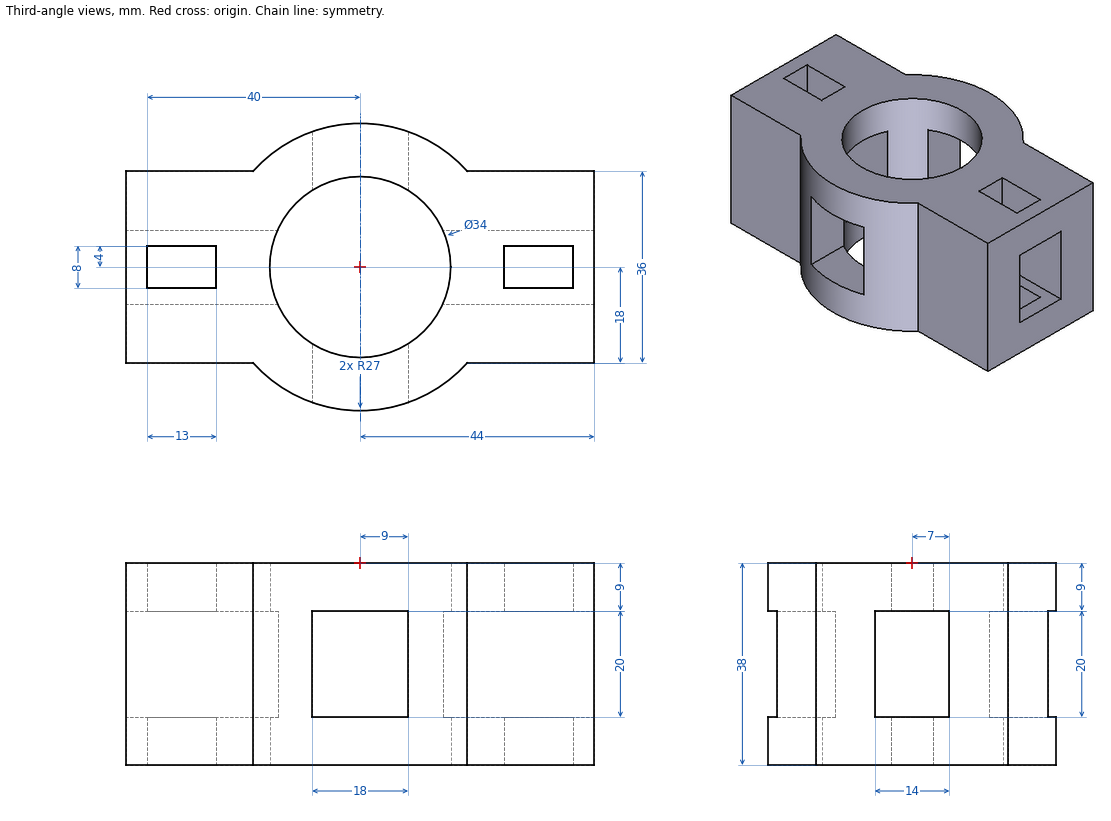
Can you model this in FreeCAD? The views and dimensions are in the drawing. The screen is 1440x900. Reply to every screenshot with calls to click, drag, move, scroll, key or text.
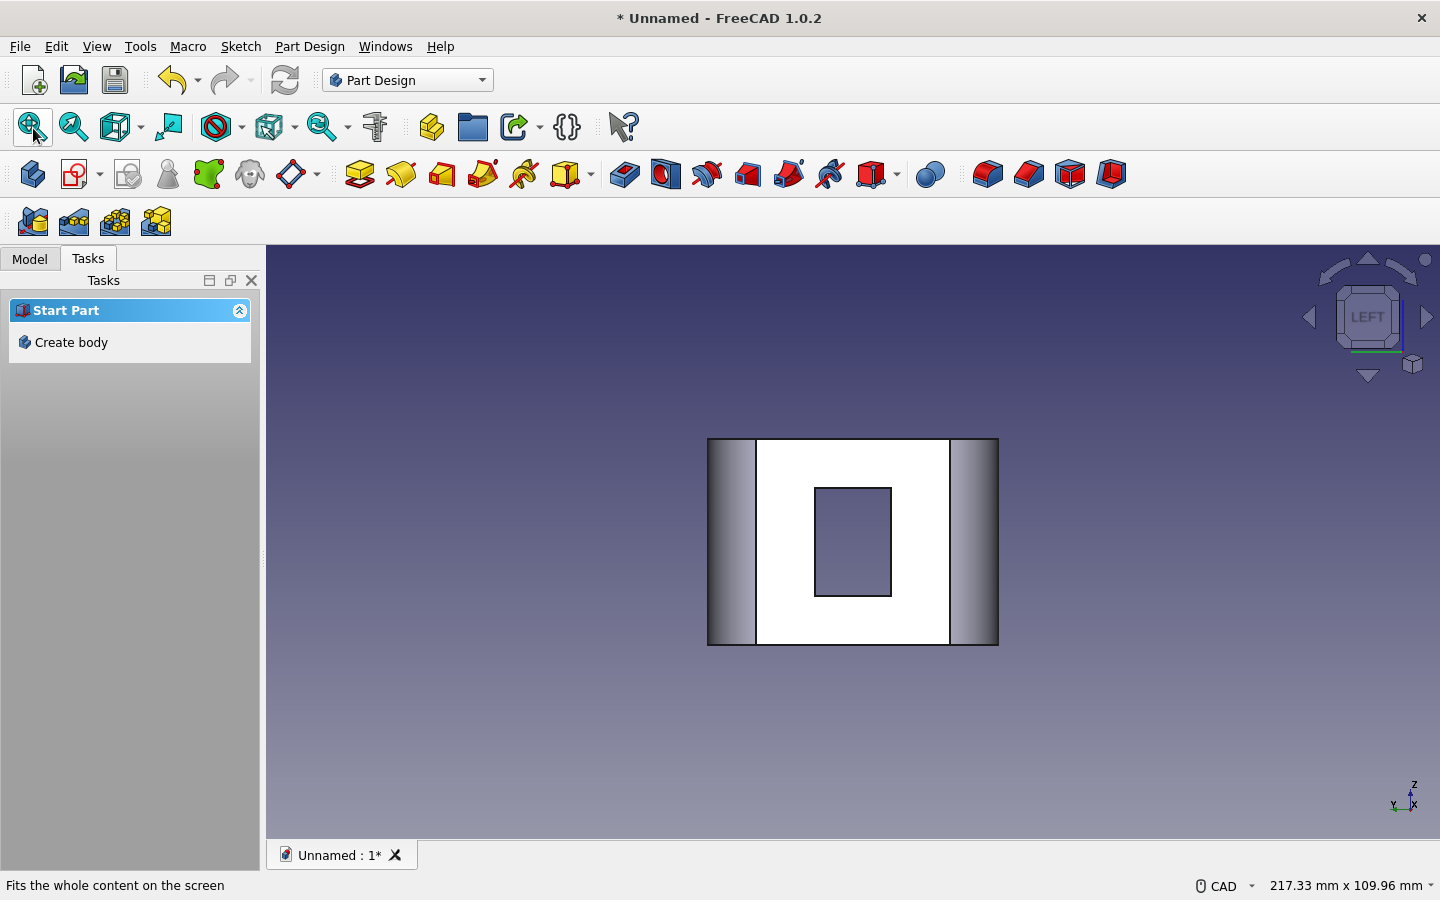
key(4)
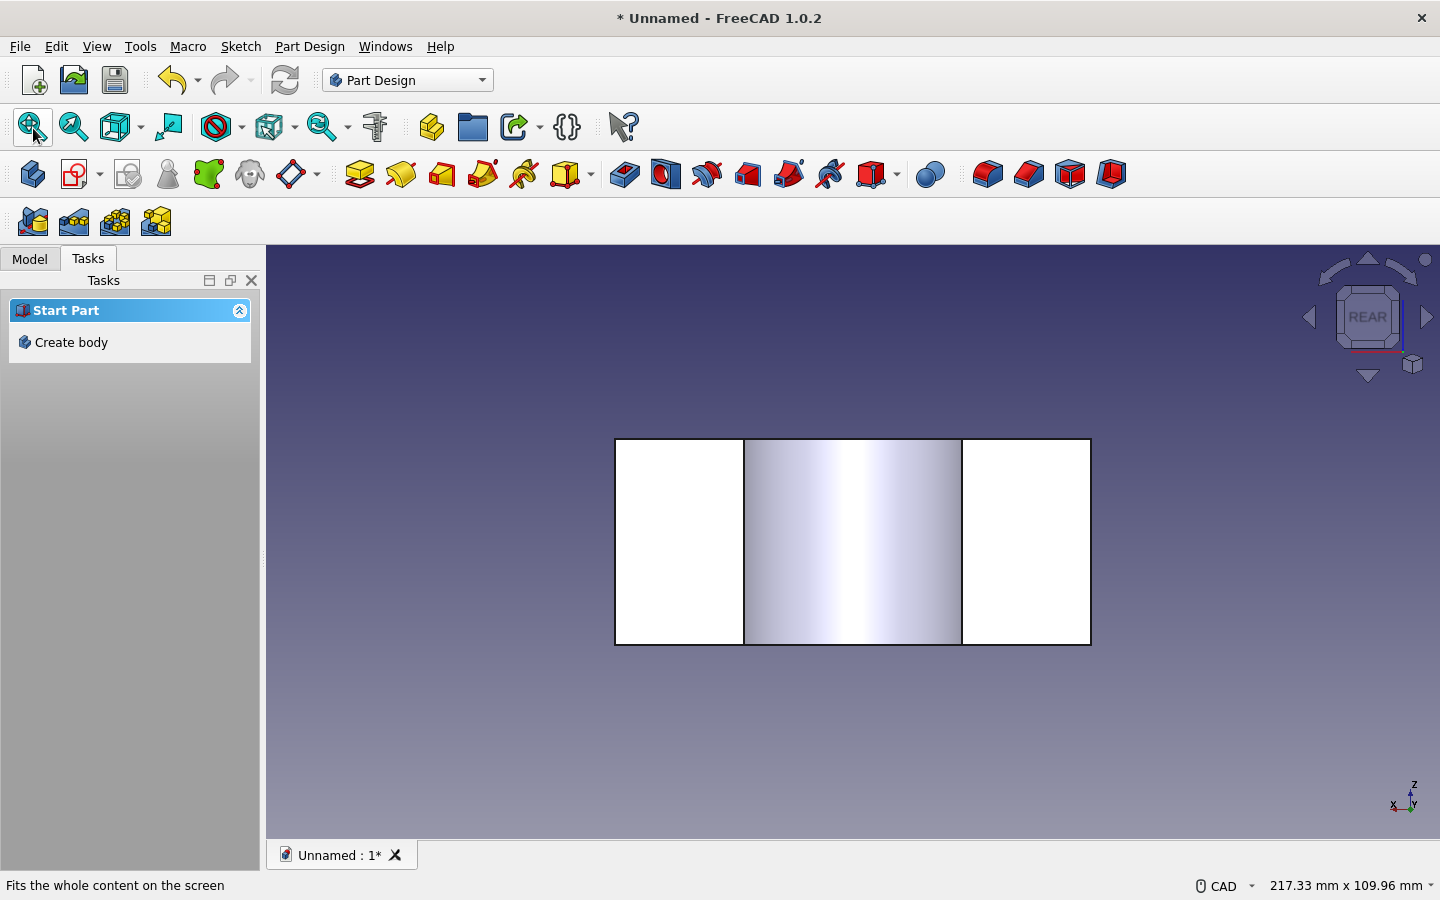
click(33, 128)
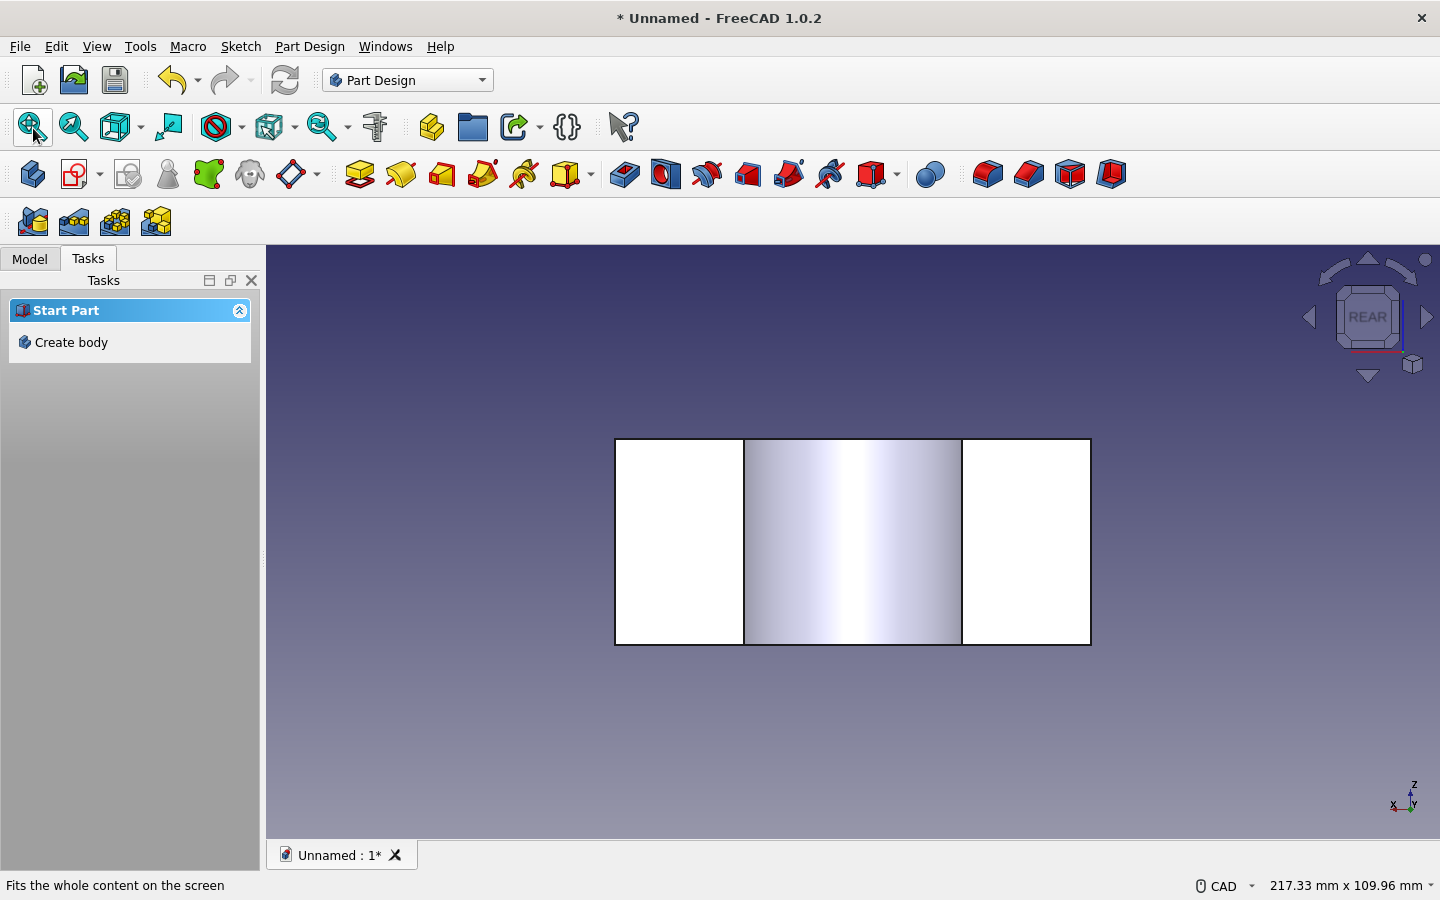
click(680, 512)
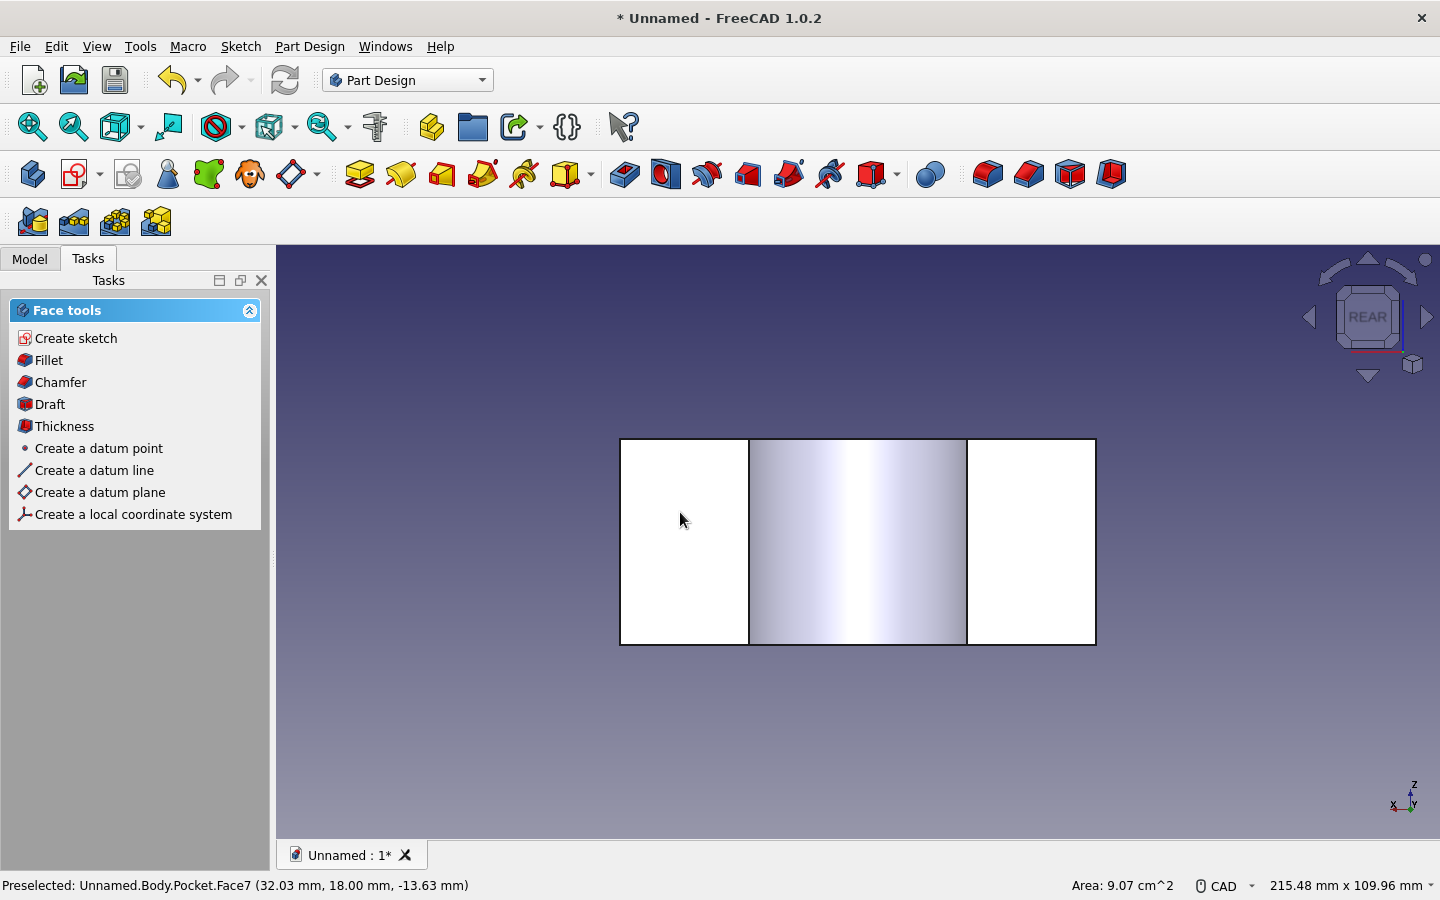
click(74, 174)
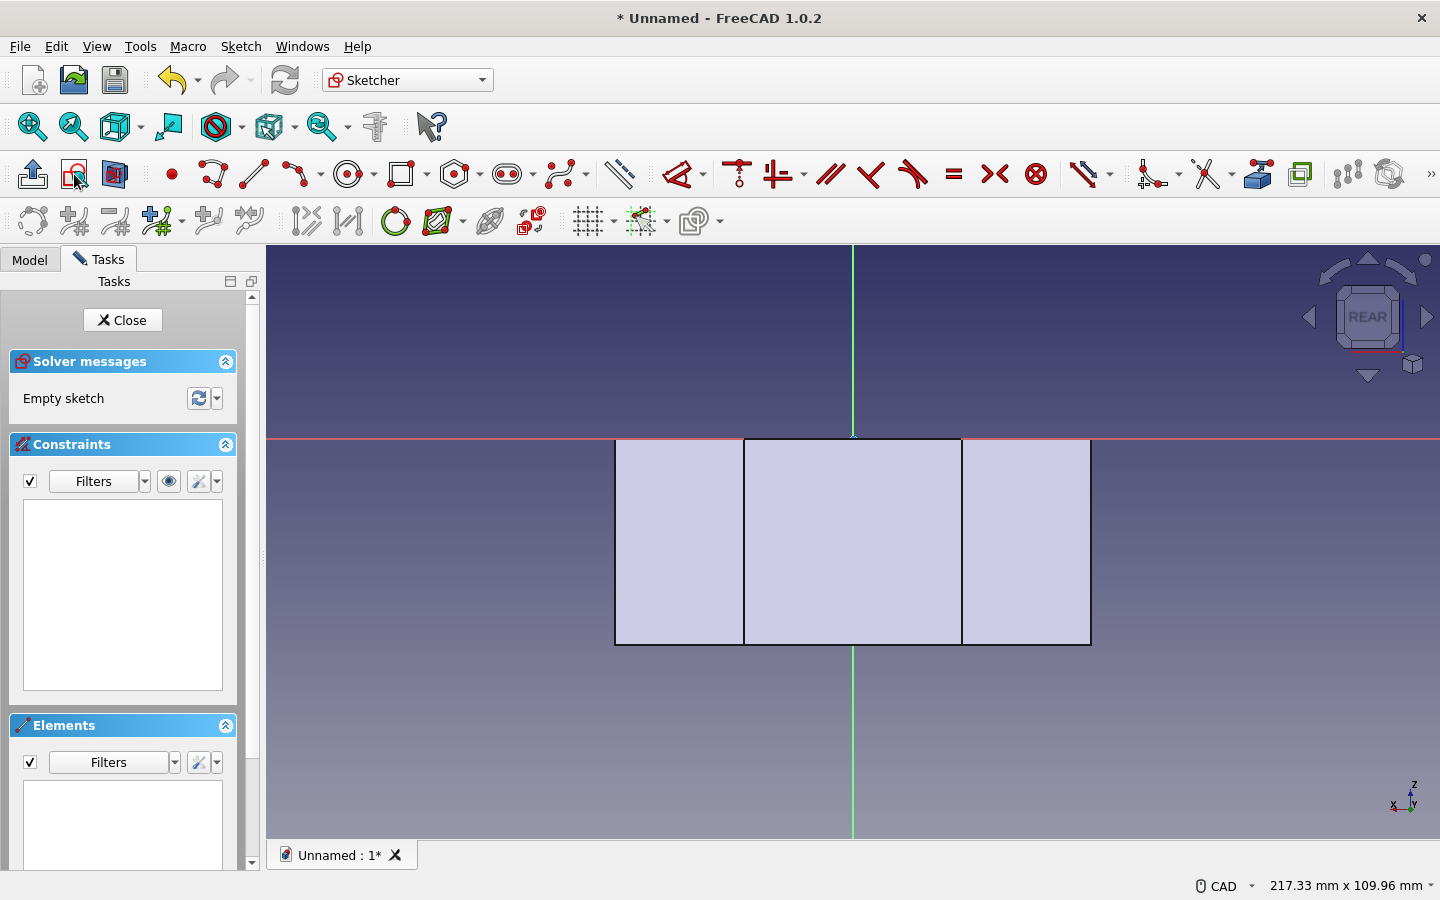
click(115, 174)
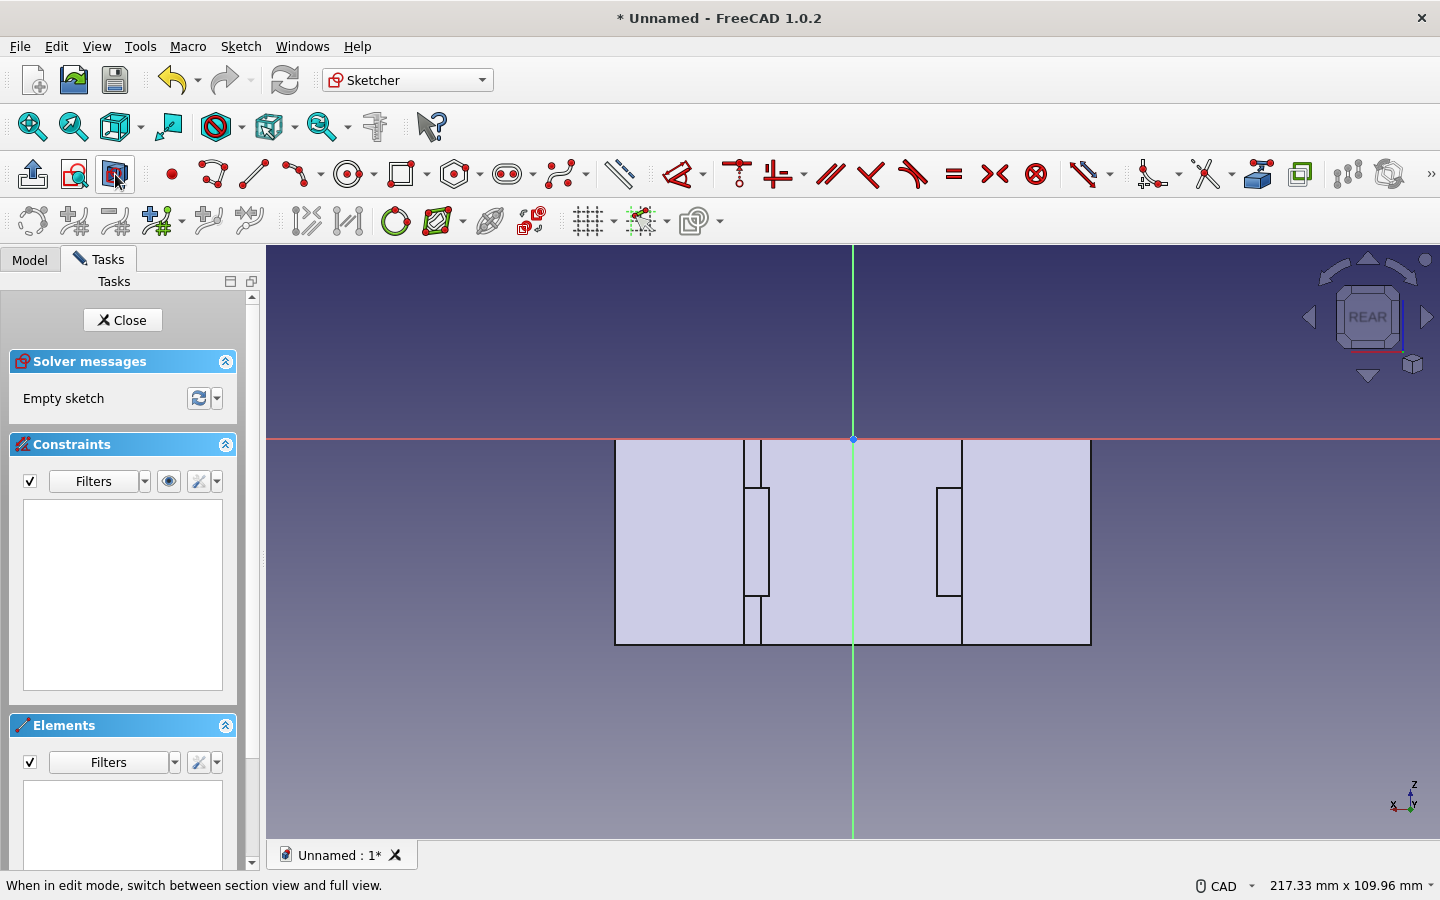
scroll(909, 498, up, 4)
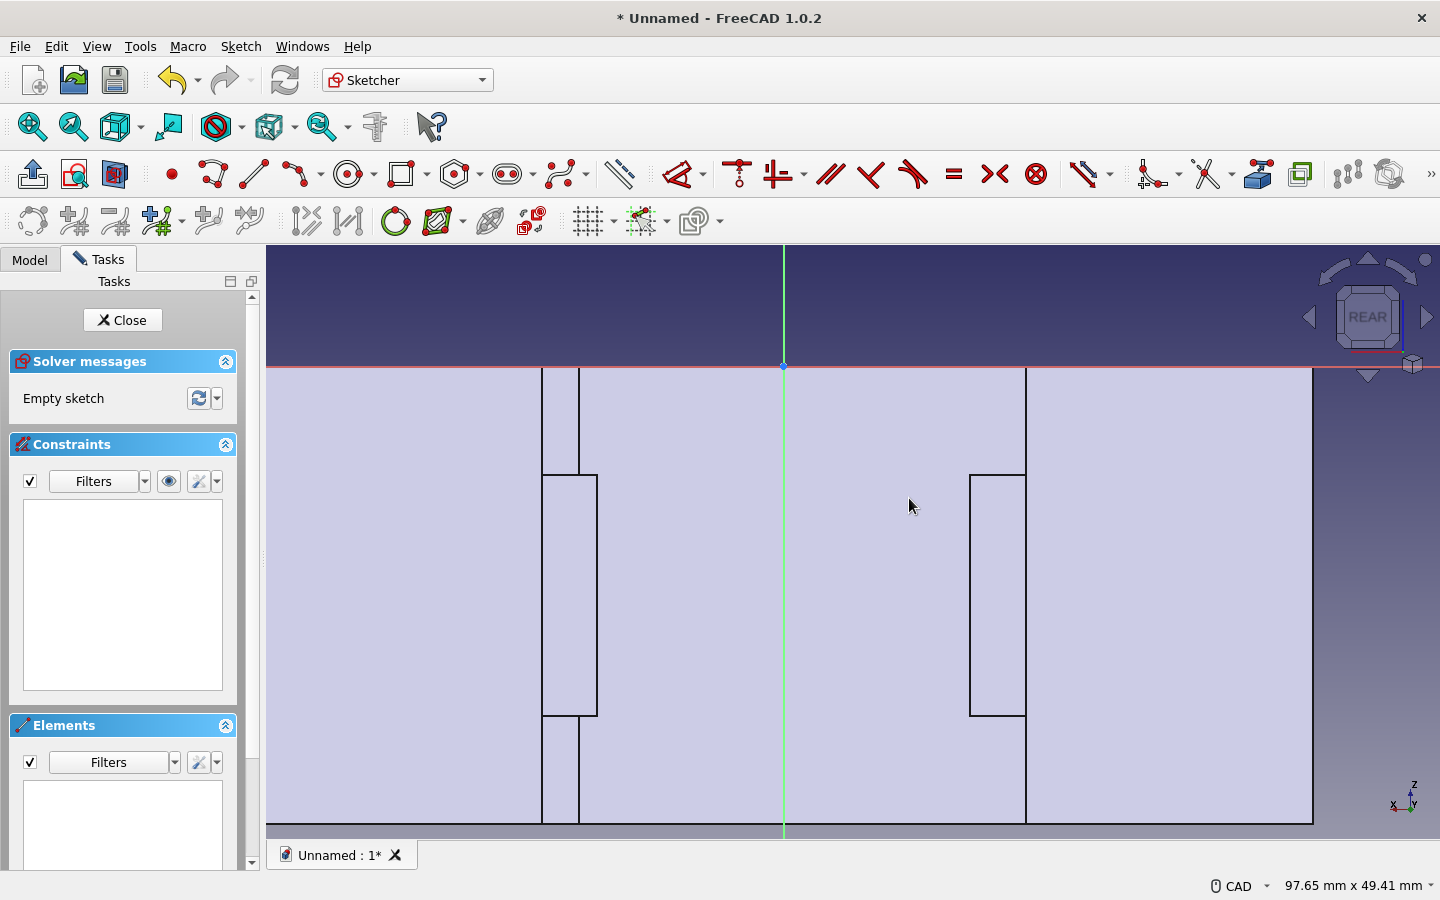
key(g)
key(r)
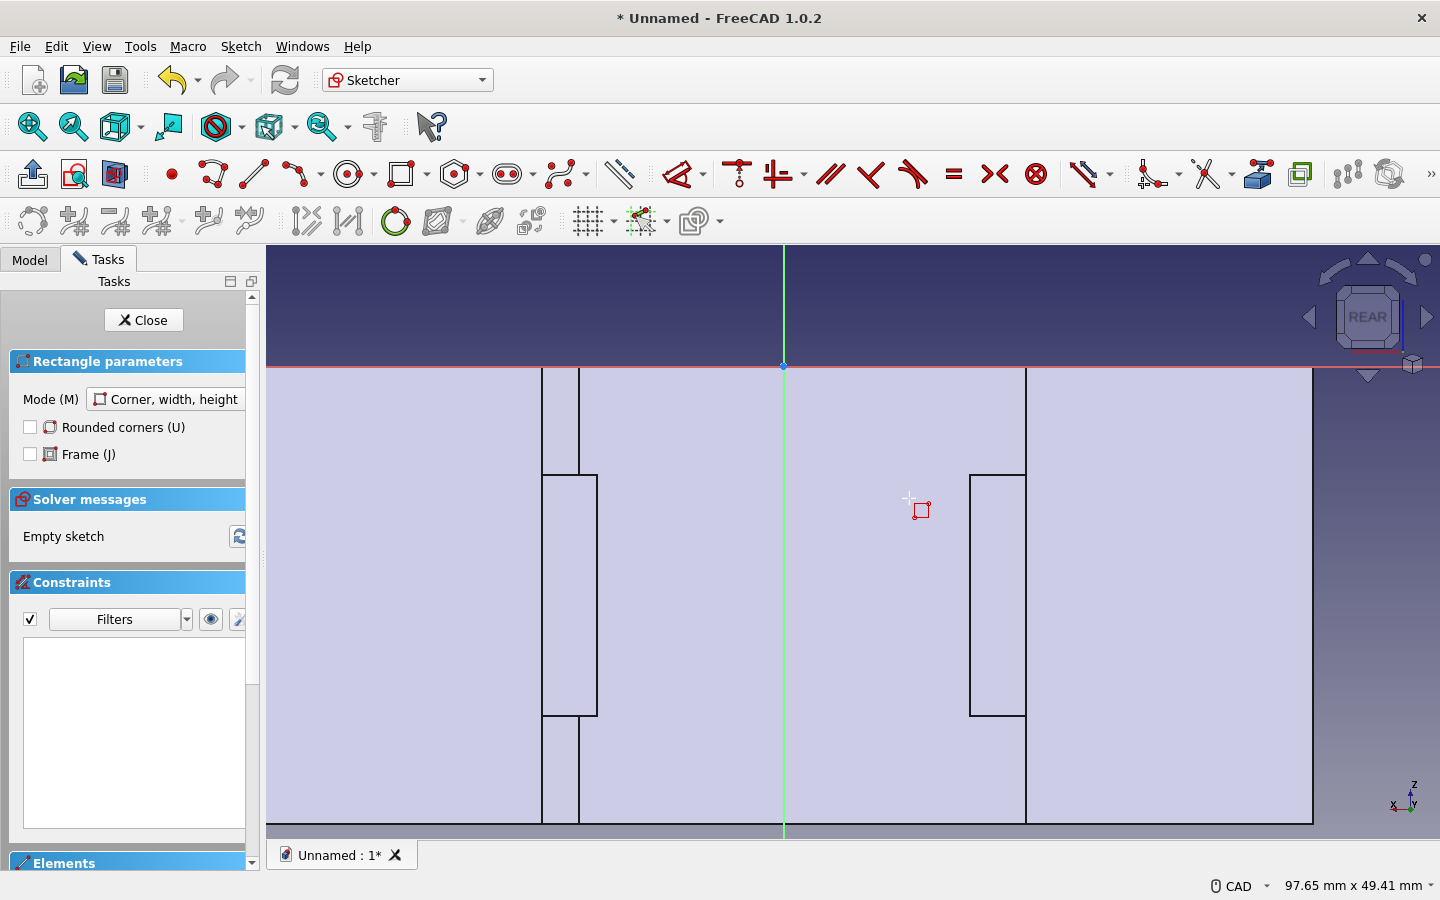
click(676, 475)
click(892, 716)
key(Escape)